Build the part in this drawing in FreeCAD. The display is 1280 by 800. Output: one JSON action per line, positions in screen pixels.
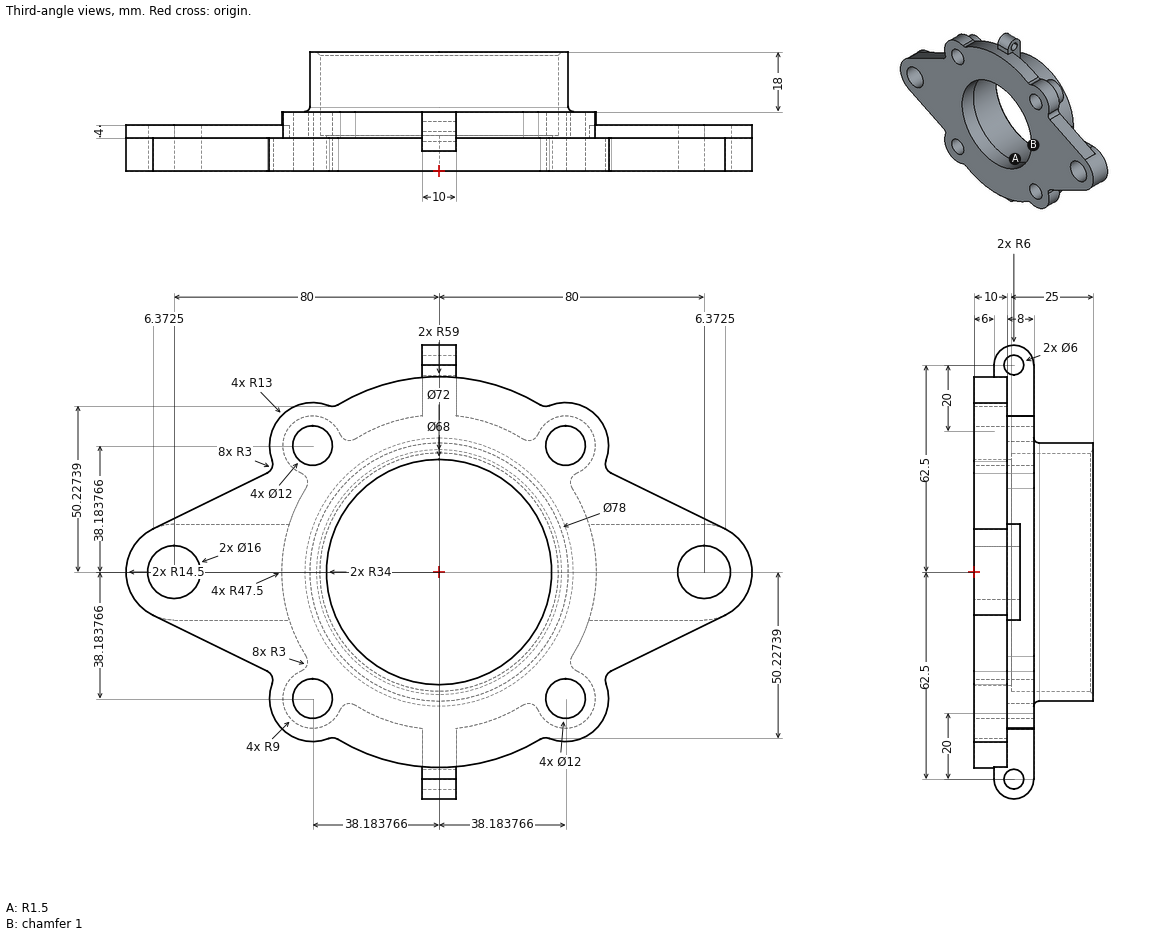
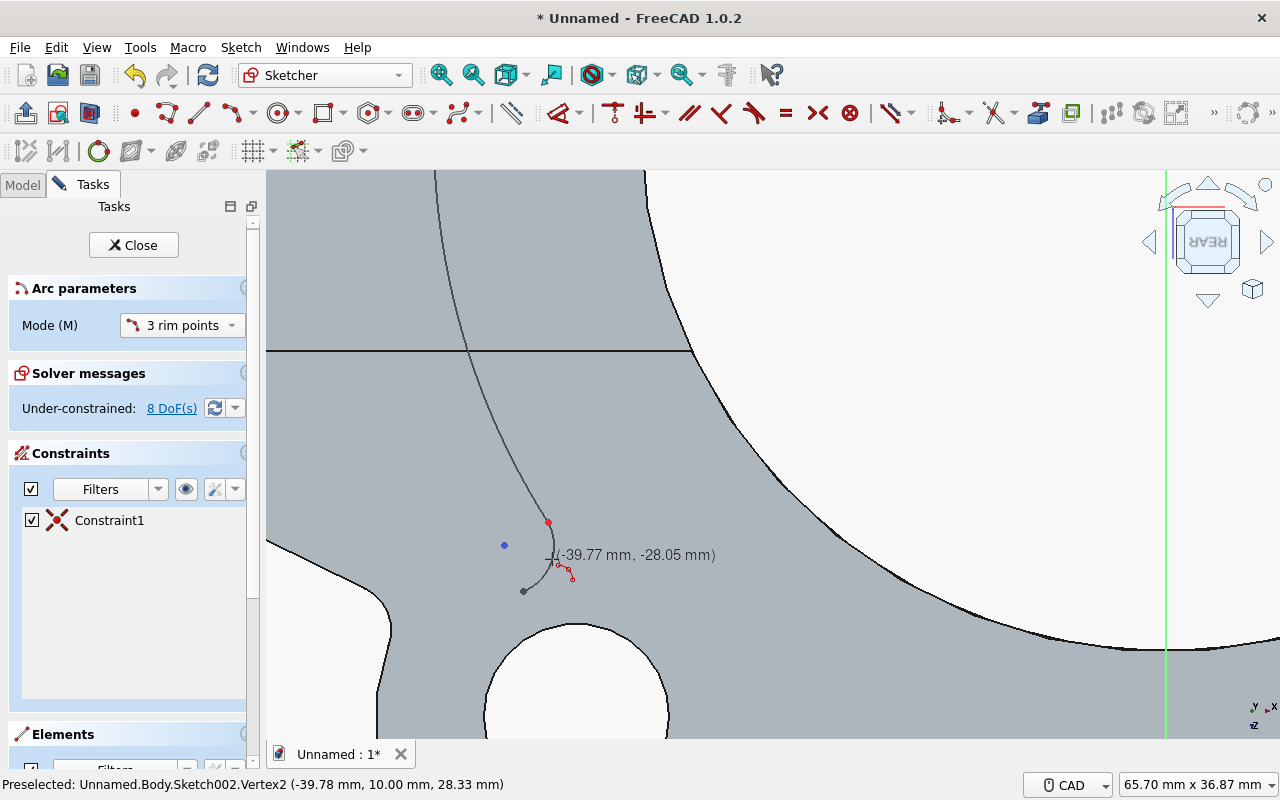
{"action": "scroll", "coordinate": [554, 562], "scroll_direction": "down", "scroll_amount": 7}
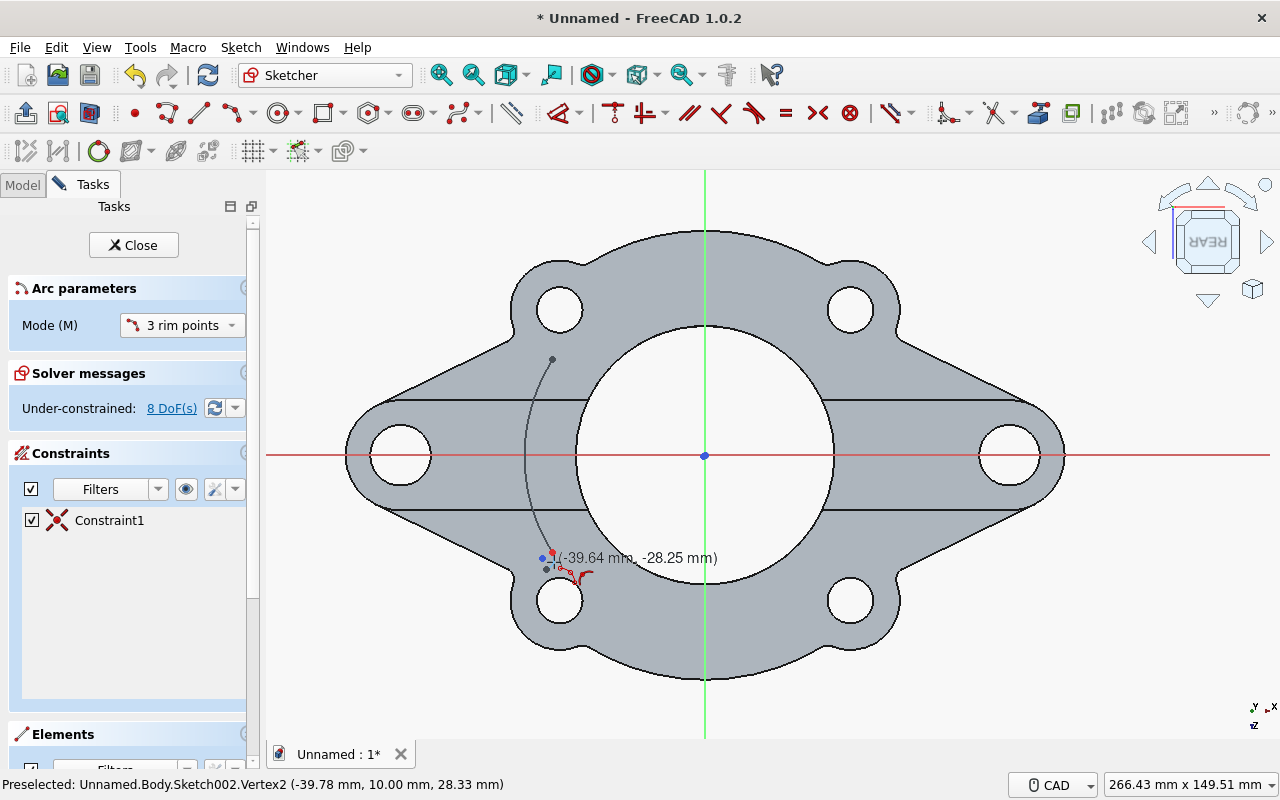
{"action": "scroll", "coordinate": [547, 569], "scroll_direction": "up", "scroll_amount": 2}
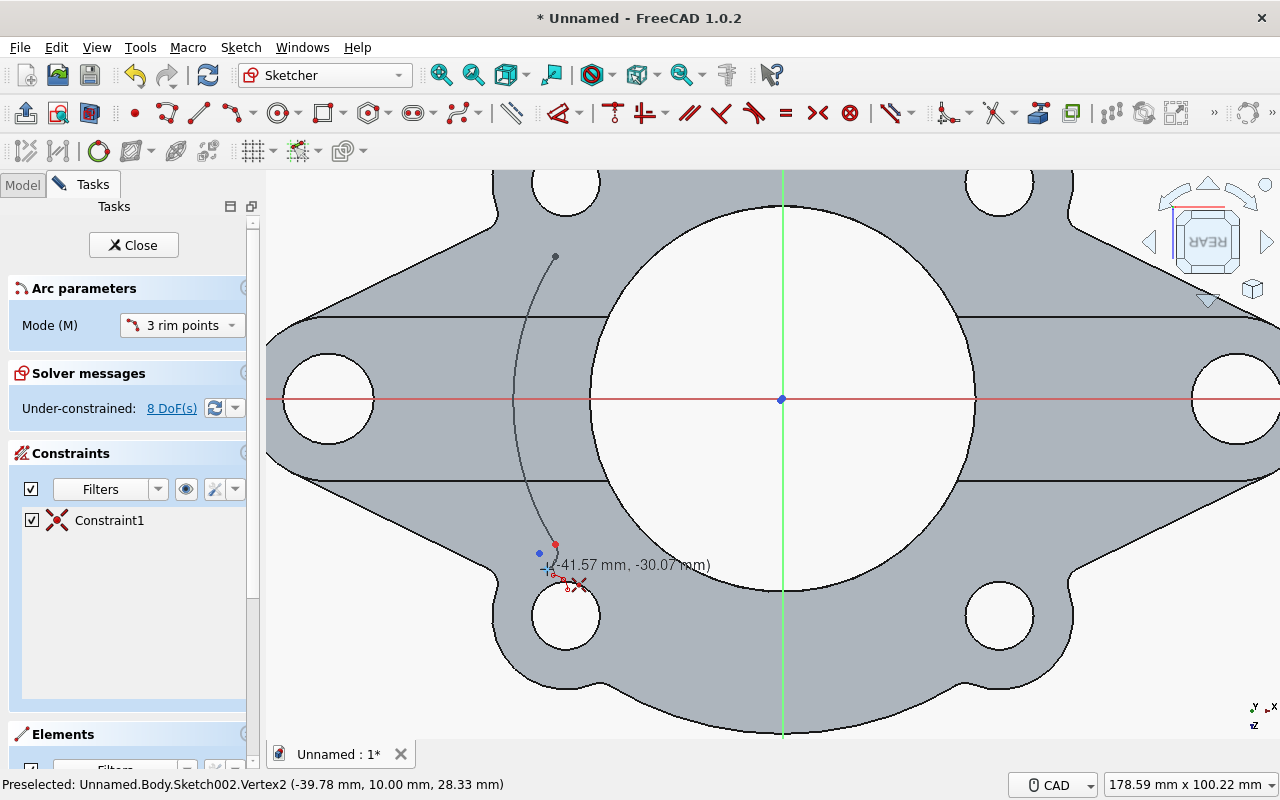
{"action": "left_click", "coordinate": [546, 570]}
{"action": "left_click", "coordinate": [613, 635]}
{"action": "left_click", "coordinate": [530, 652]}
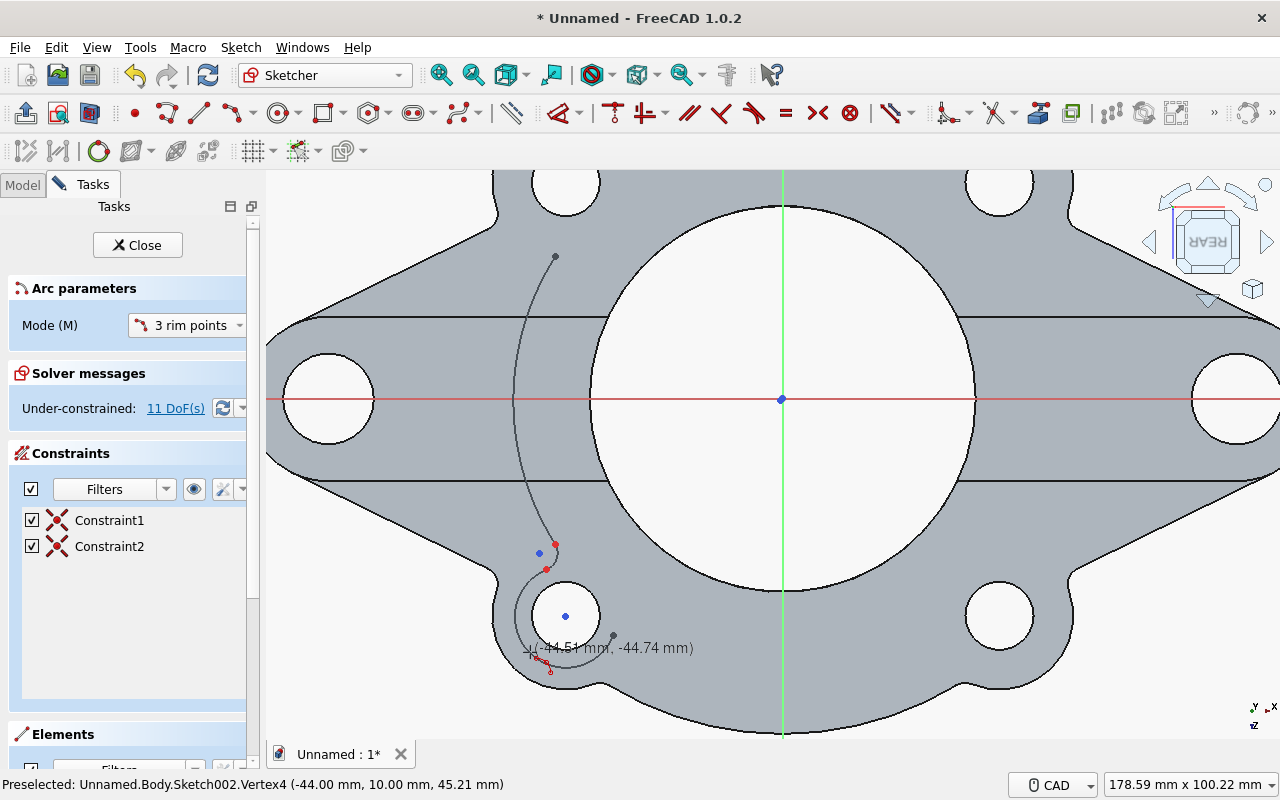
{"action": "left_click", "coordinate": [613, 636]}
{"action": "left_click", "coordinate": [638, 627]}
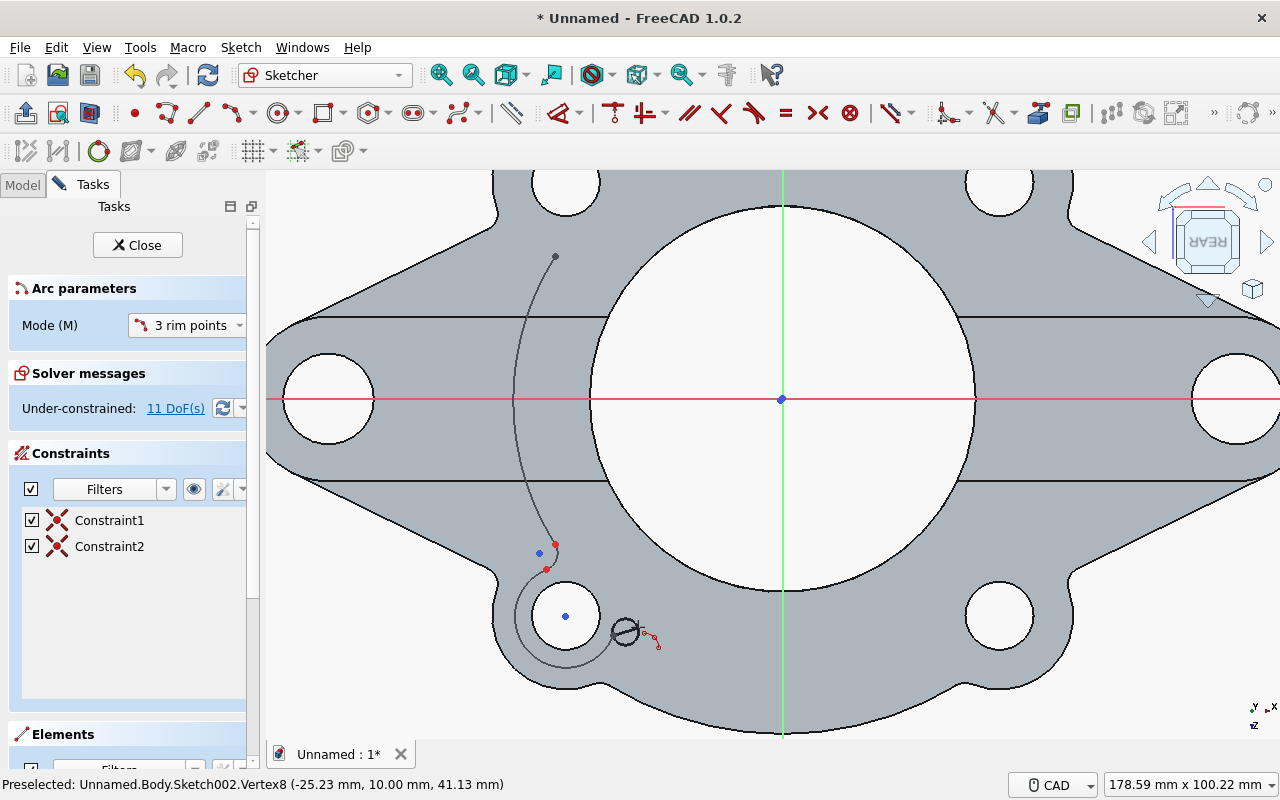
{"action": "scroll", "coordinate": [624, 625], "scroll_direction": "up", "scroll_amount": 5}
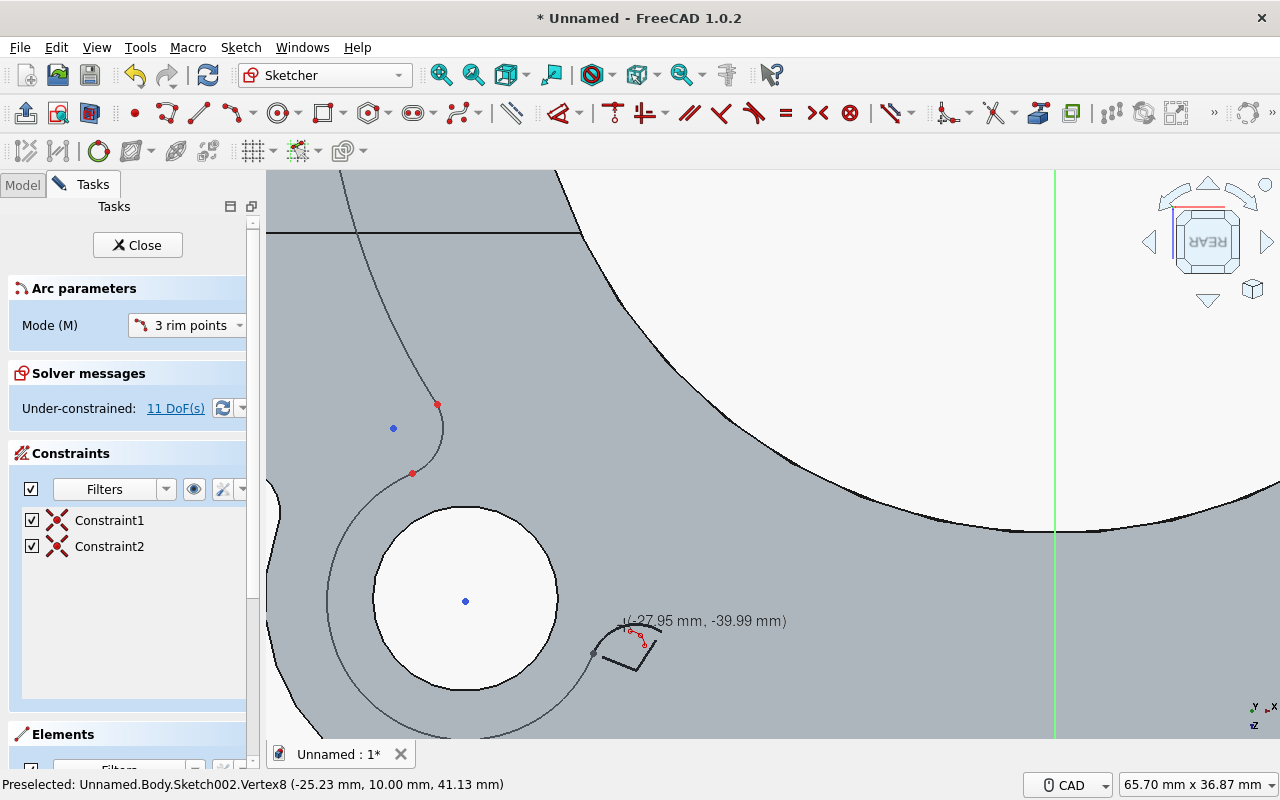
{"action": "left_click", "coordinate": [623, 623]}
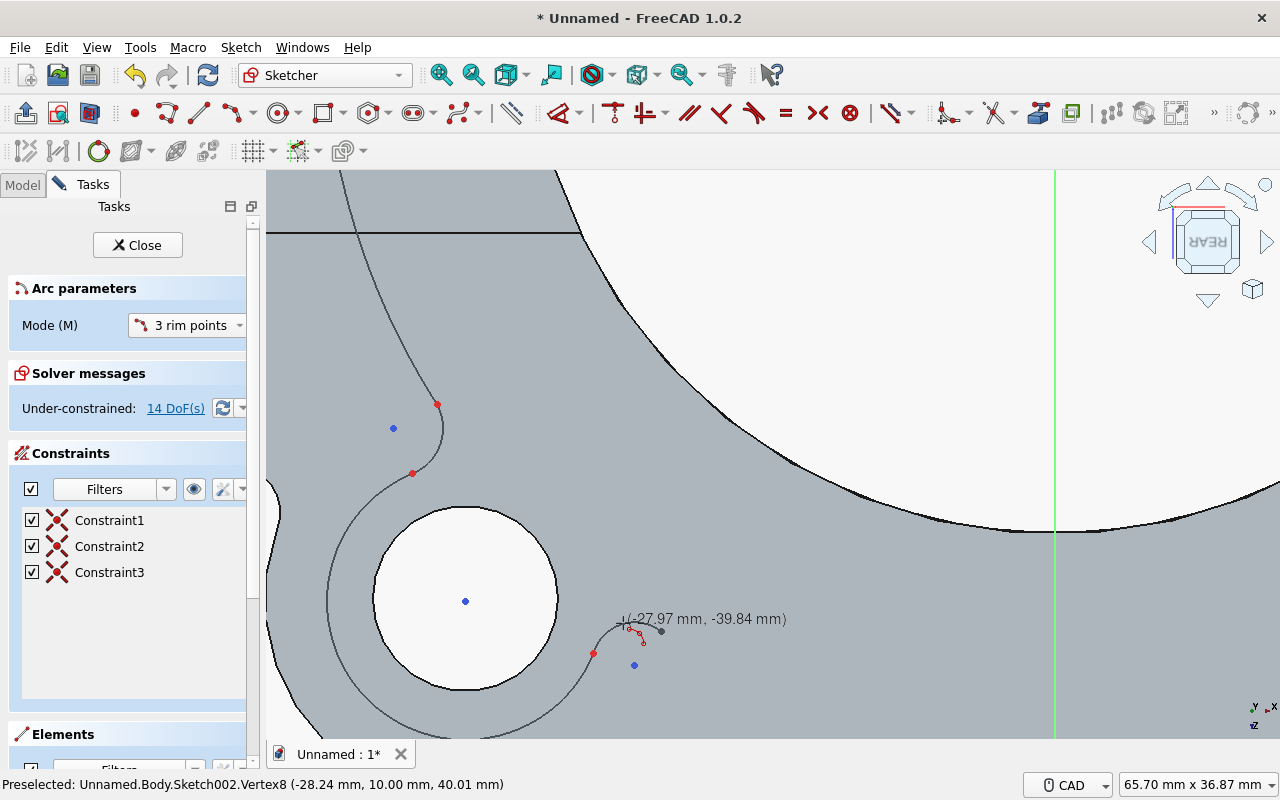
{"action": "scroll", "coordinate": [590, 600], "scroll_direction": "down", "scroll_amount": 7}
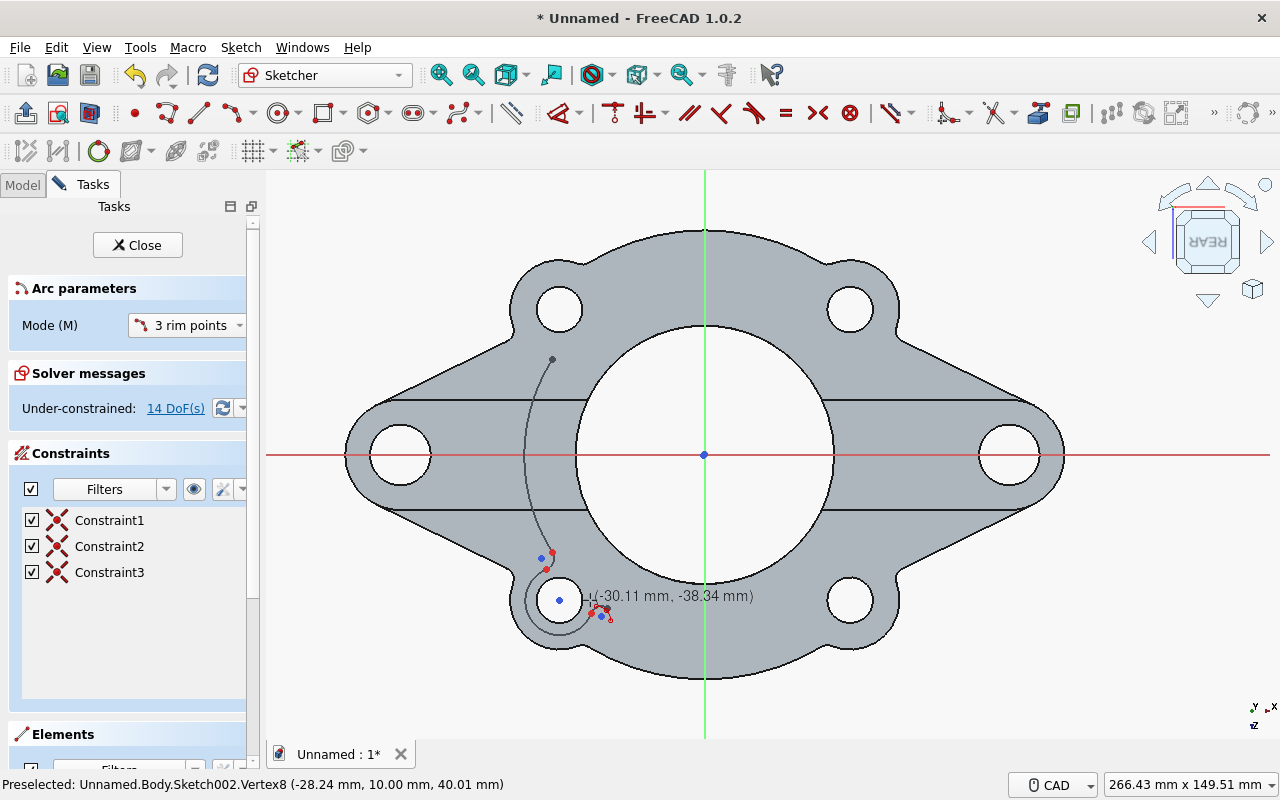
{"action": "scroll", "coordinate": [608, 608], "scroll_direction": "up", "scroll_amount": 2}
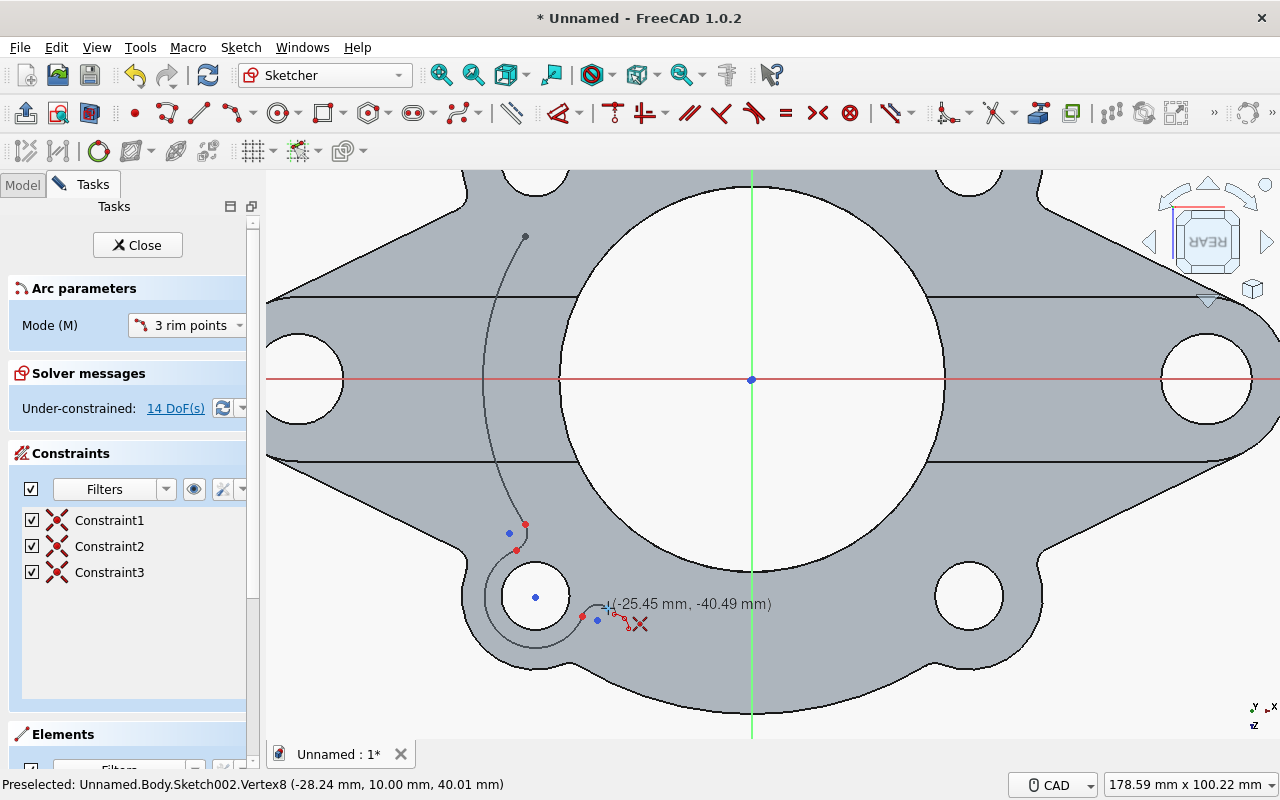
{"action": "left_click", "coordinate": [608, 608]}
{"action": "left_click", "coordinate": [897, 607]}
{"action": "left_click", "coordinate": [722, 647]}